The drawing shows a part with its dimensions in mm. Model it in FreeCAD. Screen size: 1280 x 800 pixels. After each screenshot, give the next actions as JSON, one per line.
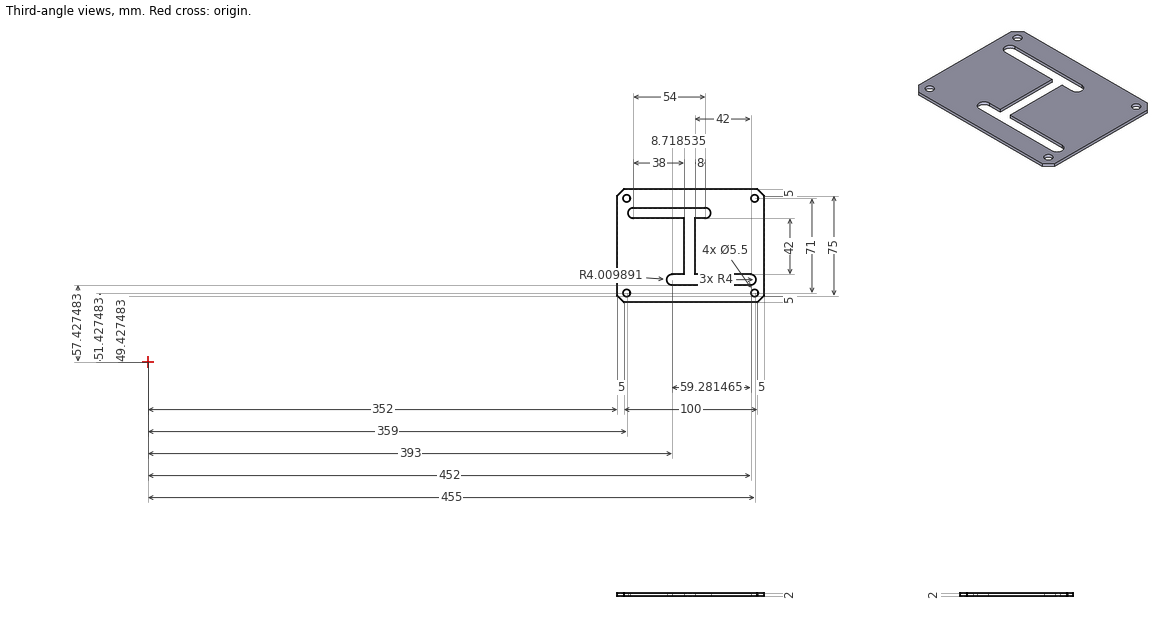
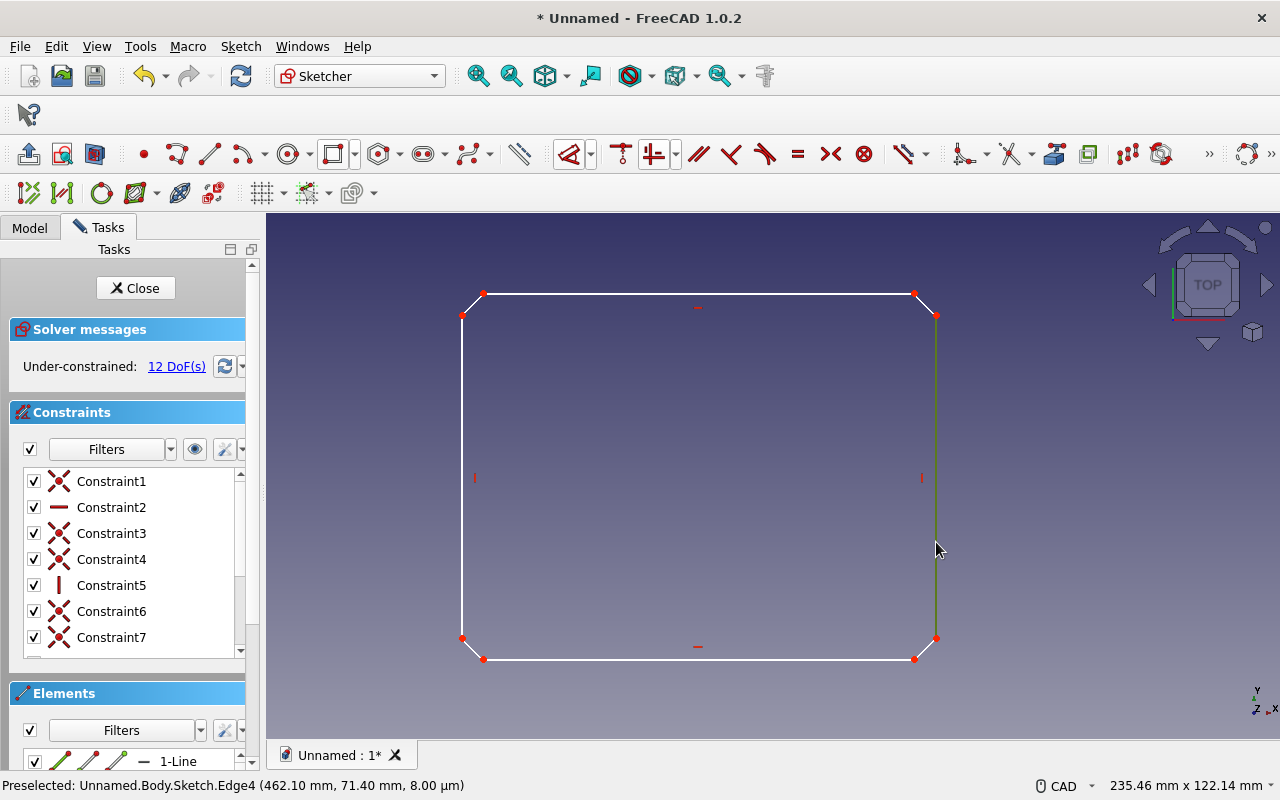
{"action": "key", "text": "i"}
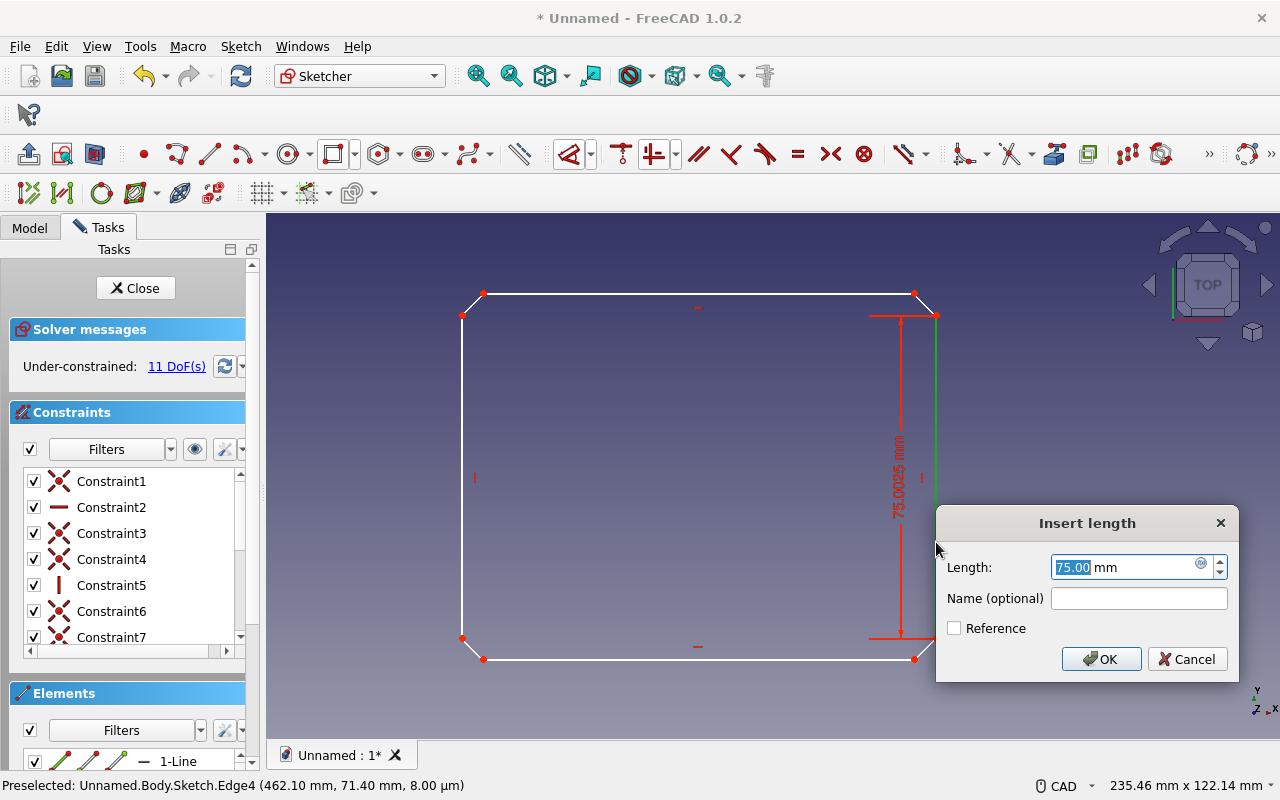
{"action": "type", "text": "75"}
{"action": "key", "text": "Return"}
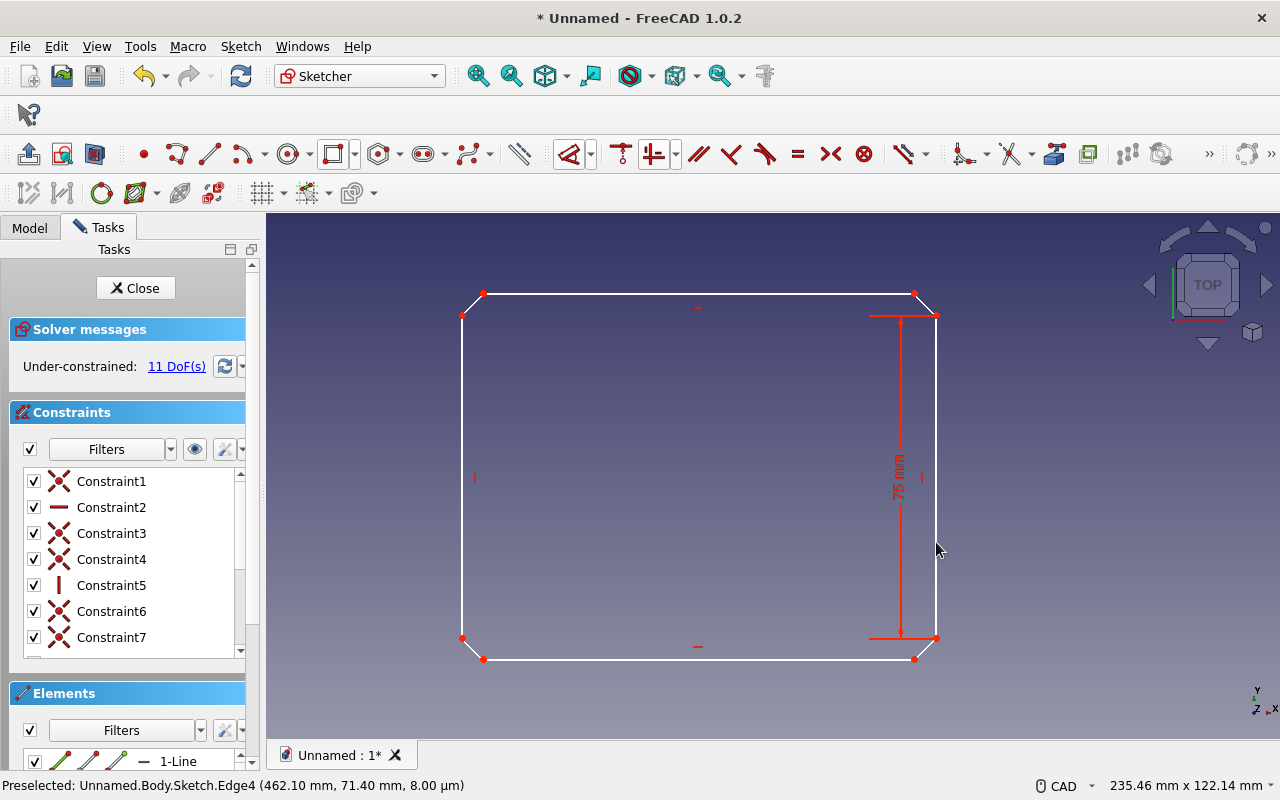
{"action": "left_click", "coordinate": [462, 413]}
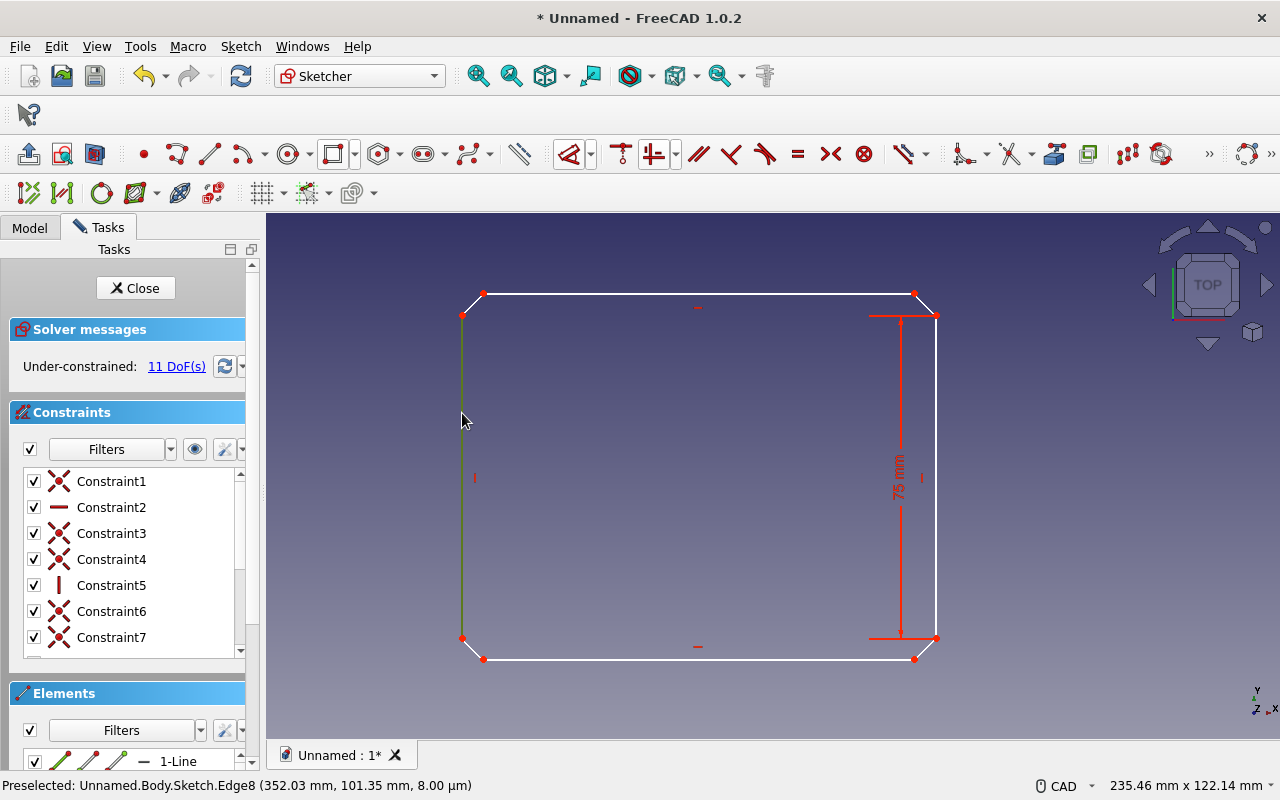
{"action": "key", "text": "i"}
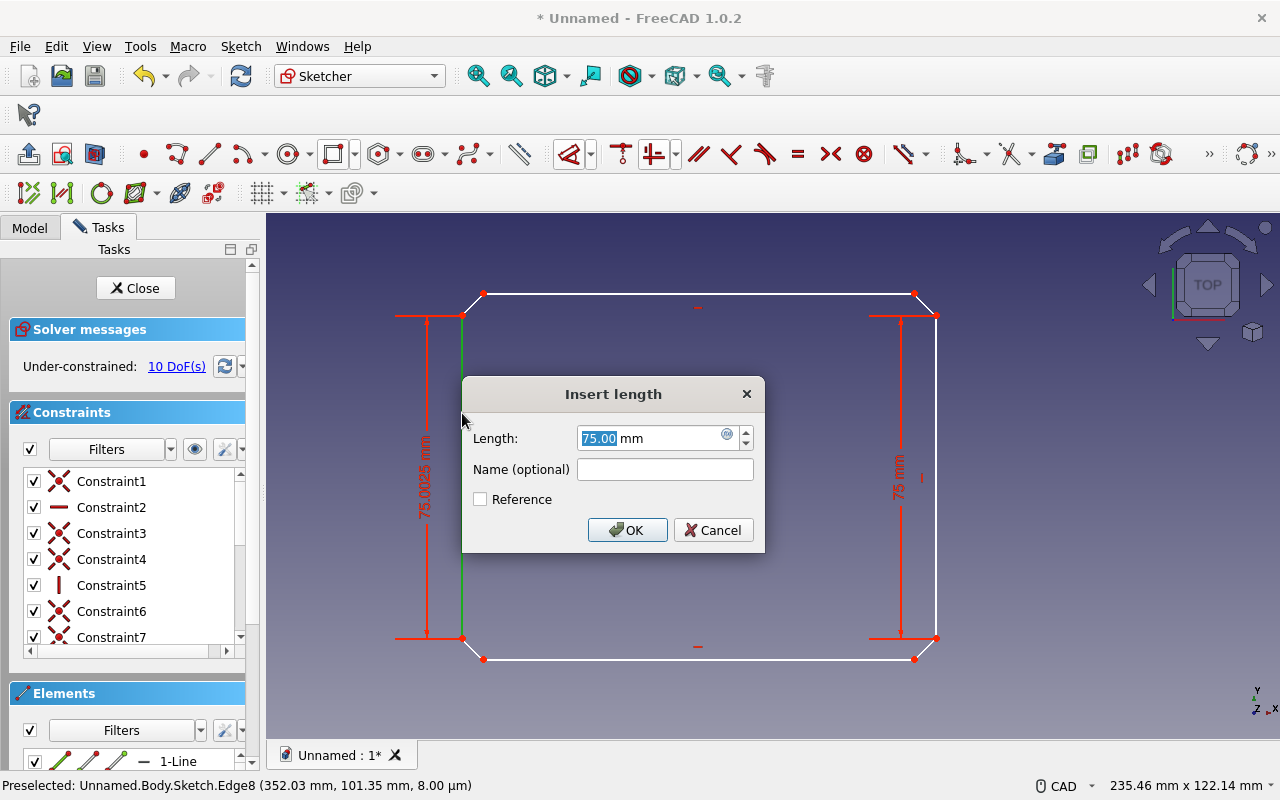
{"action": "type", "text": "75"}
{"action": "key", "text": "Return"}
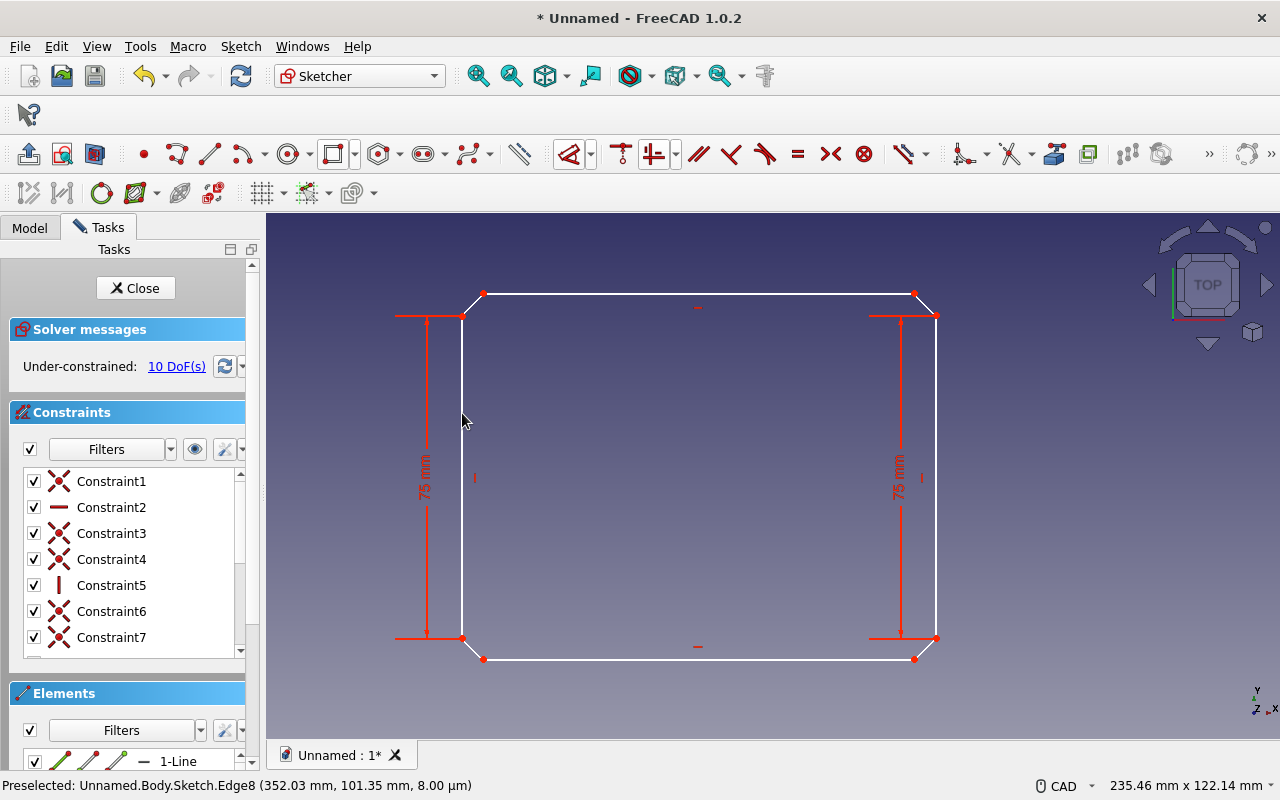
{"action": "scroll", "coordinate": [470, 647], "scroll_direction": "up", "scroll_amount": 4}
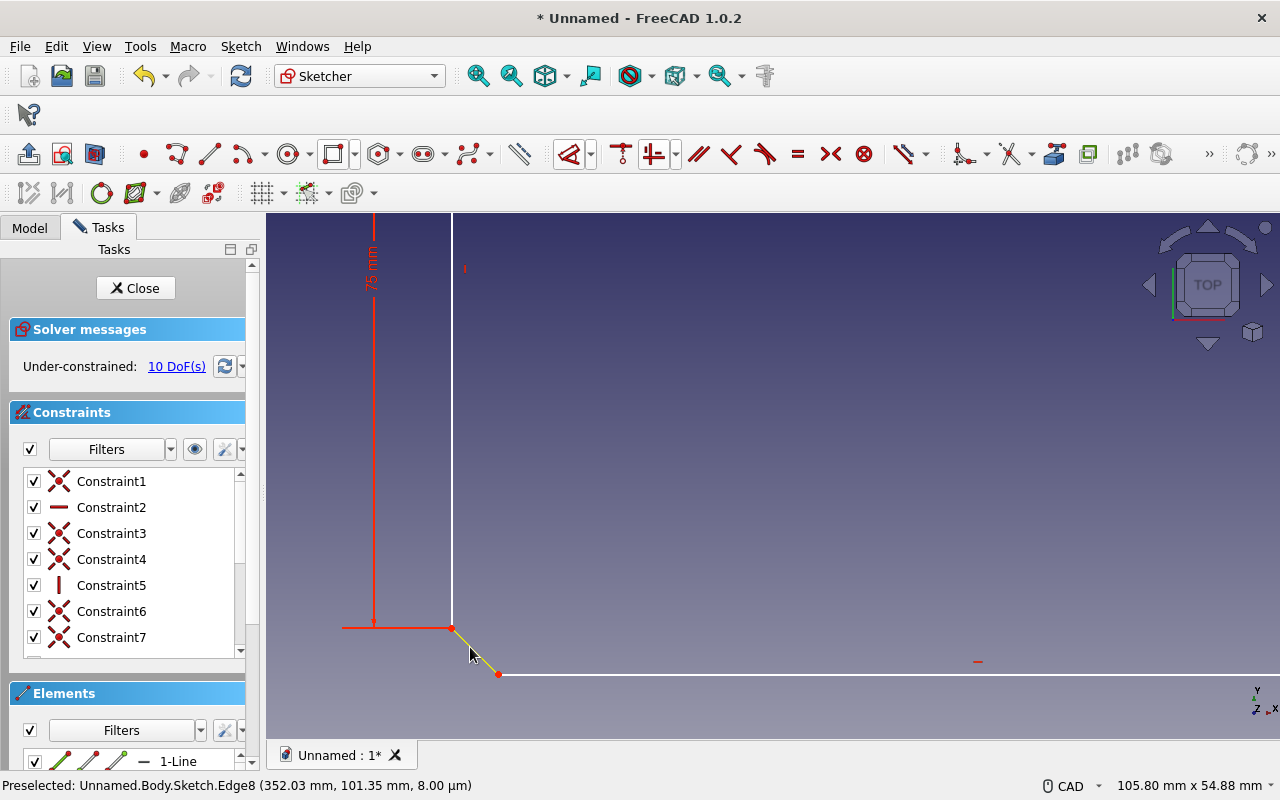
{"action": "left_click", "coordinate": [471, 647]}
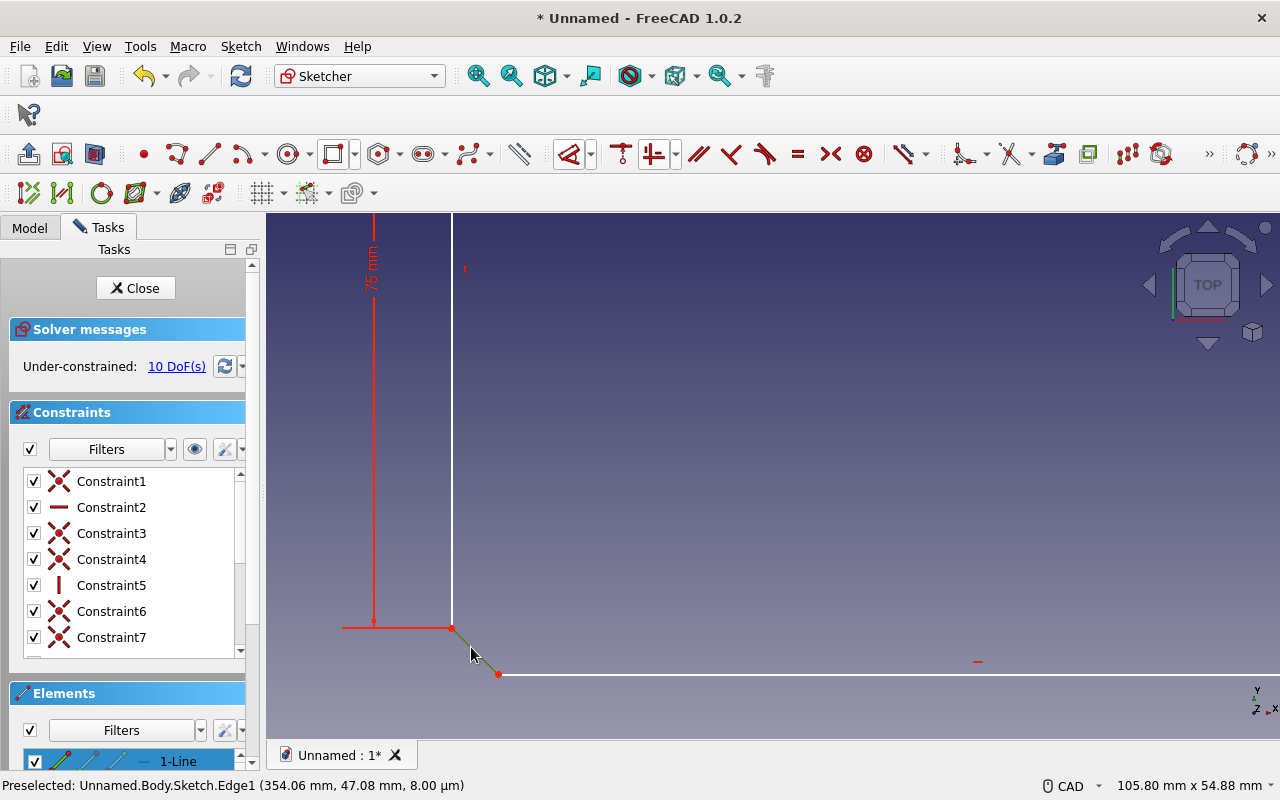
{"action": "left_click", "coordinate": [590, 154]}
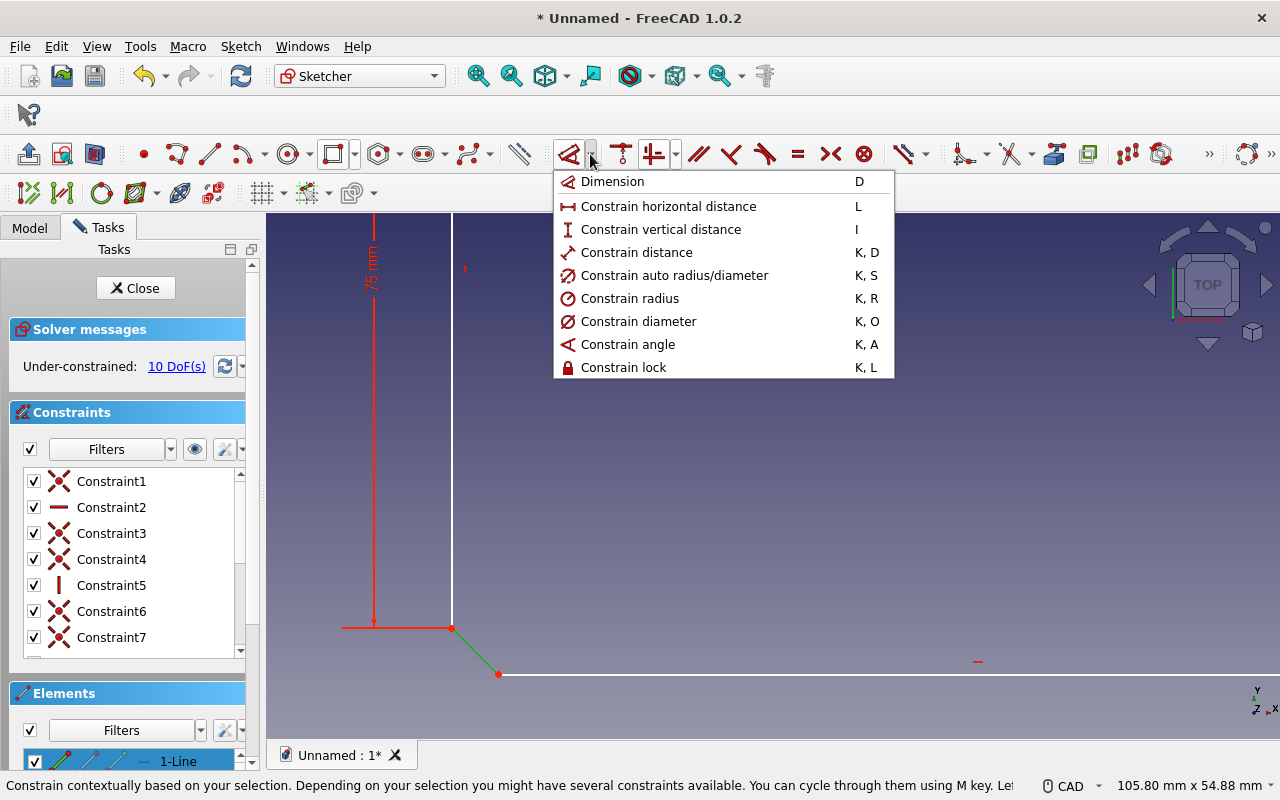
{"action": "left_click", "coordinate": [724, 206]}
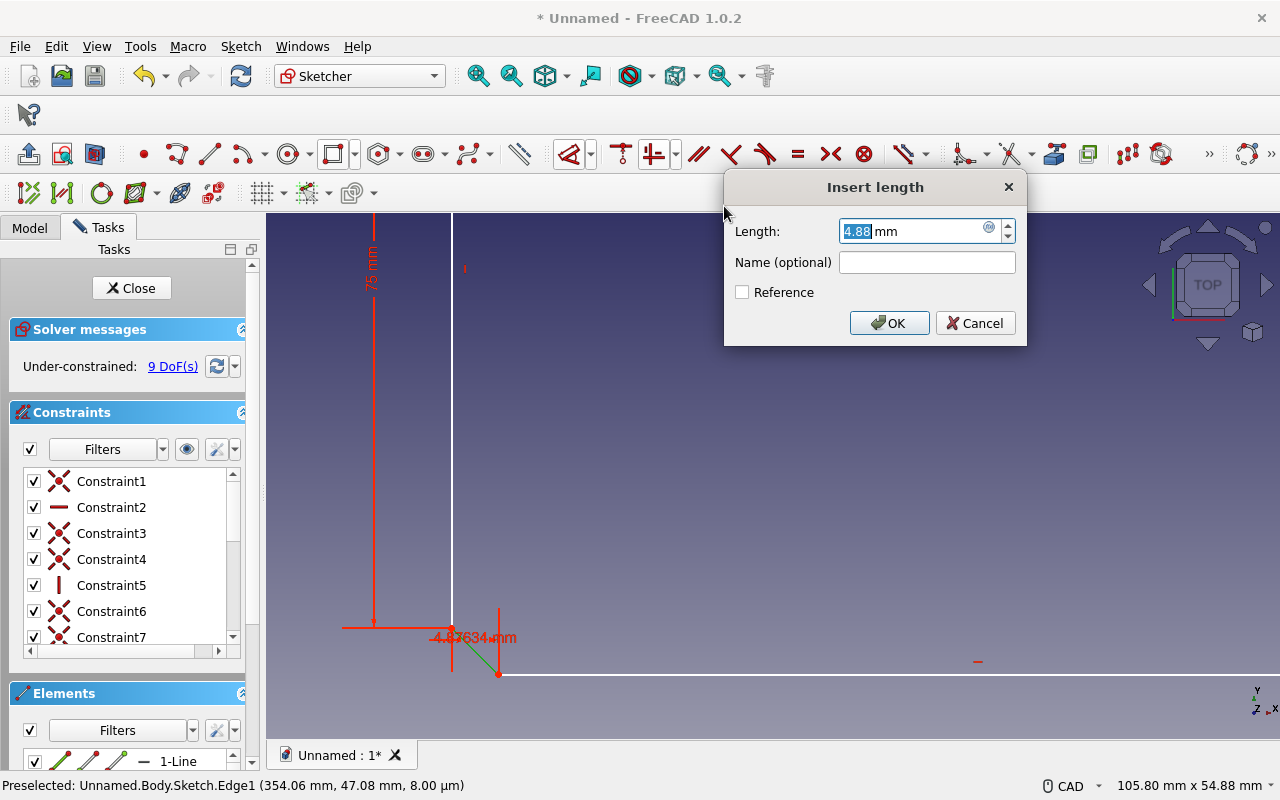
{"action": "type", "text": "5"}
{"action": "key", "text": "Return"}